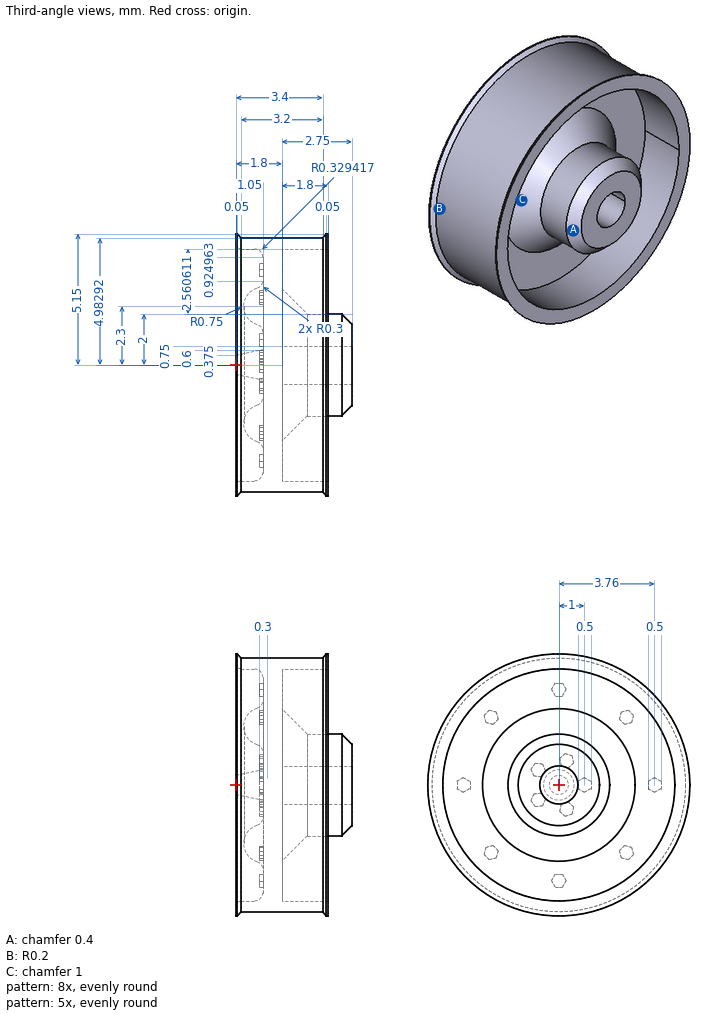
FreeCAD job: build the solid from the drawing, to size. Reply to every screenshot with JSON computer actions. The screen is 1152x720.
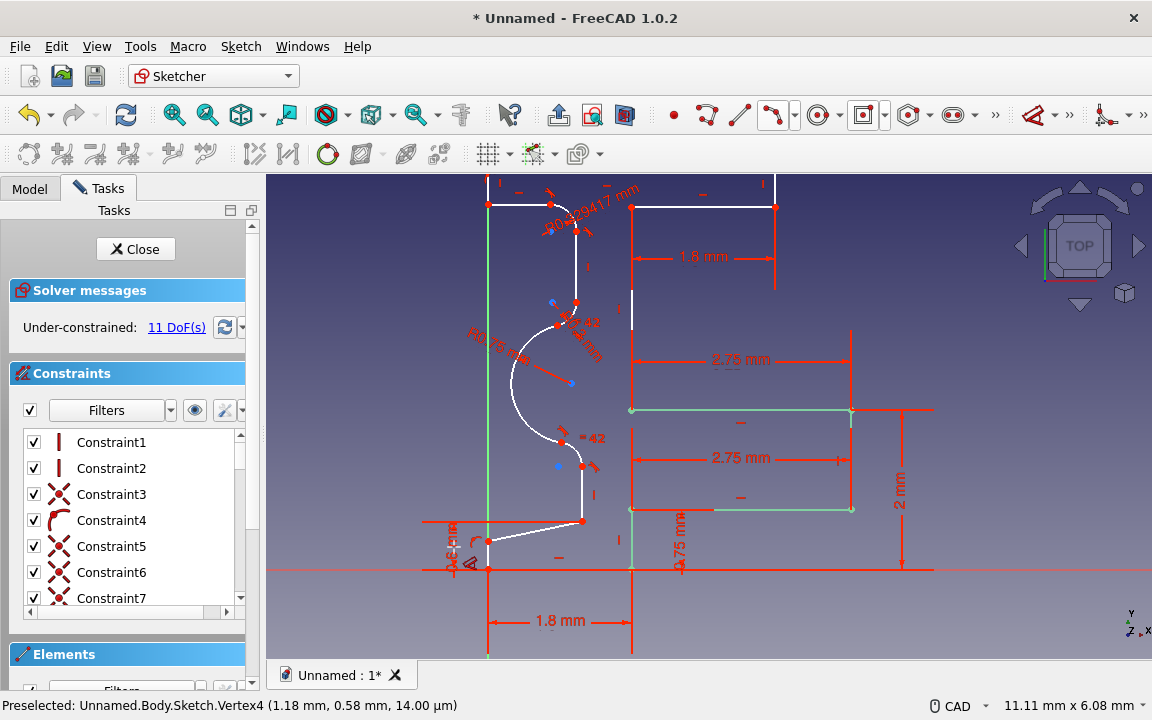
{"action": "scroll", "coordinate": [581, 523], "scroll_direction": "down", "scroll_amount": 2}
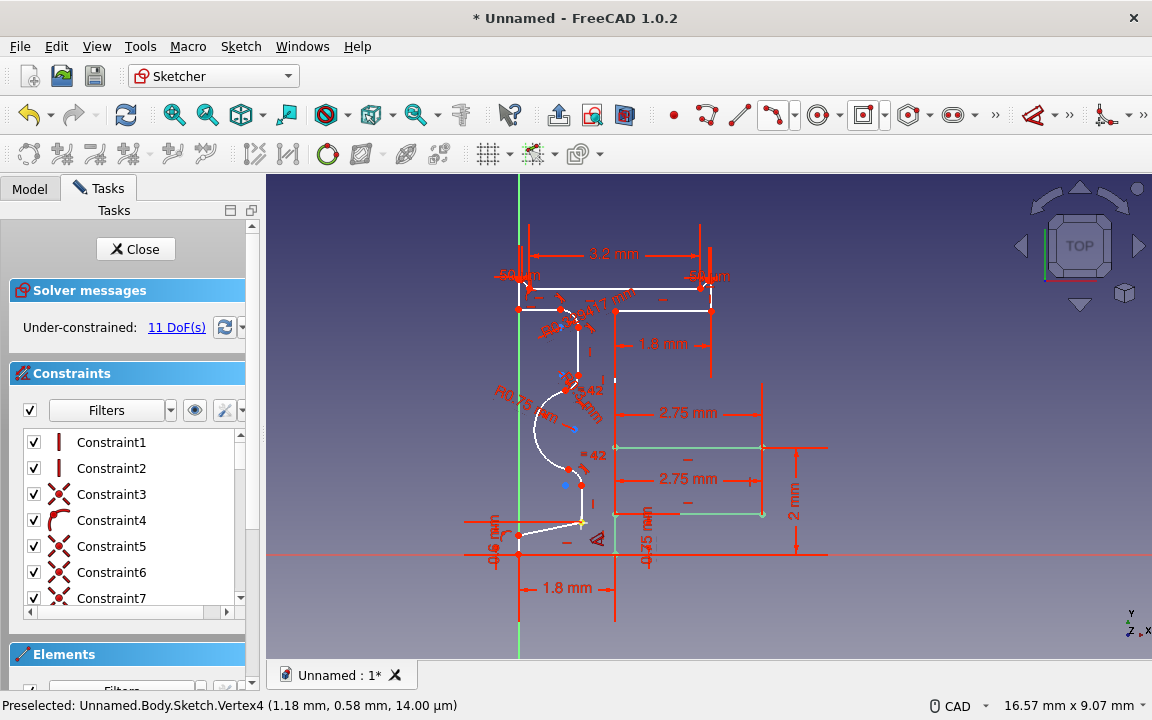
{"action": "left_click", "coordinate": [700, 289]}
{"action": "left_click", "coordinate": [651, 589]}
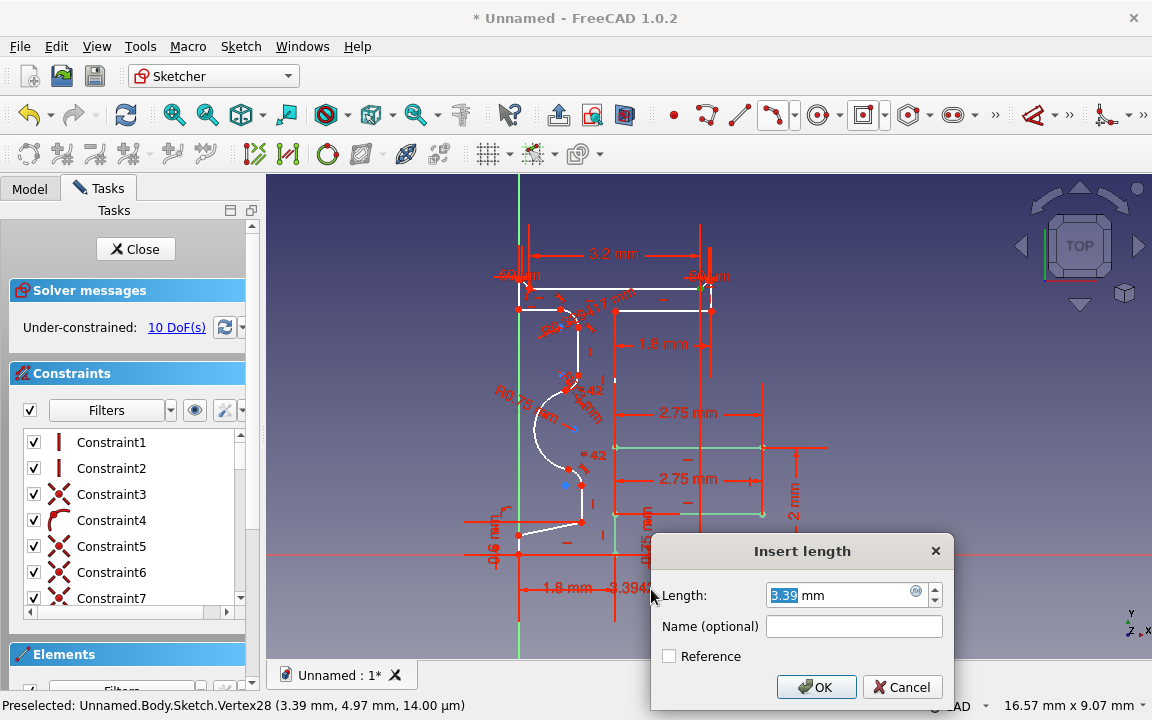
{"action": "type", "text": "3.4"}
{"action": "key", "text": "Return"}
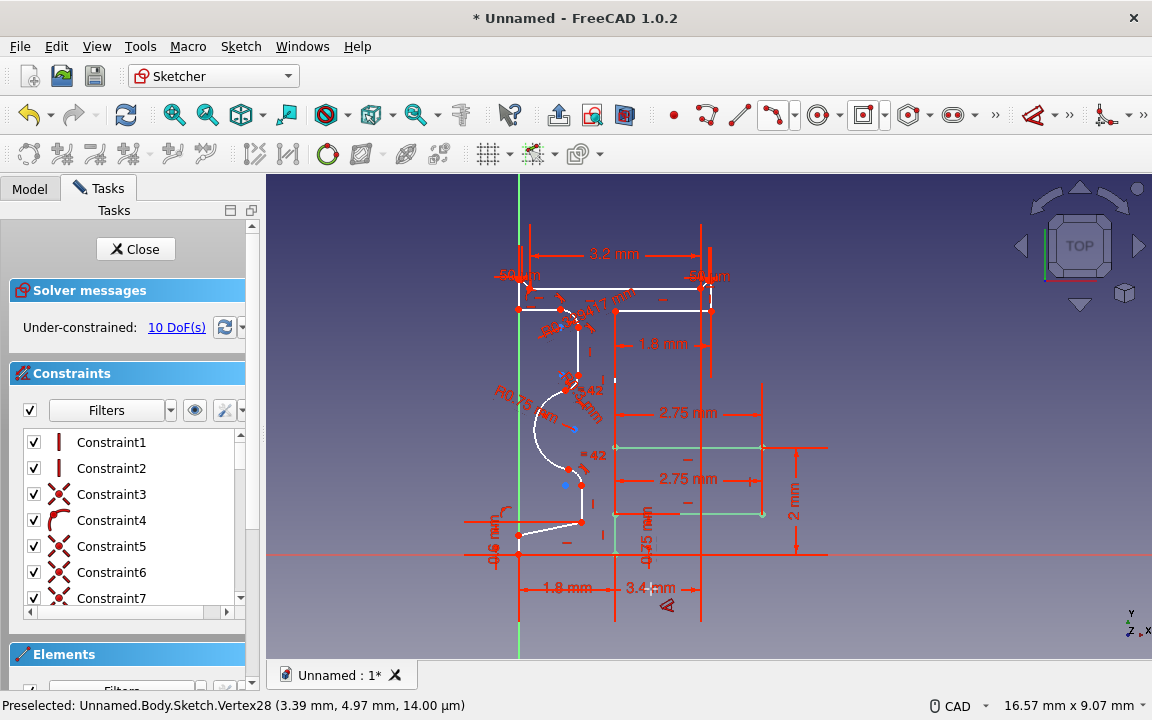
{"action": "left_click", "coordinate": [574, 430]}
{"action": "left_click", "coordinate": [485, 492]}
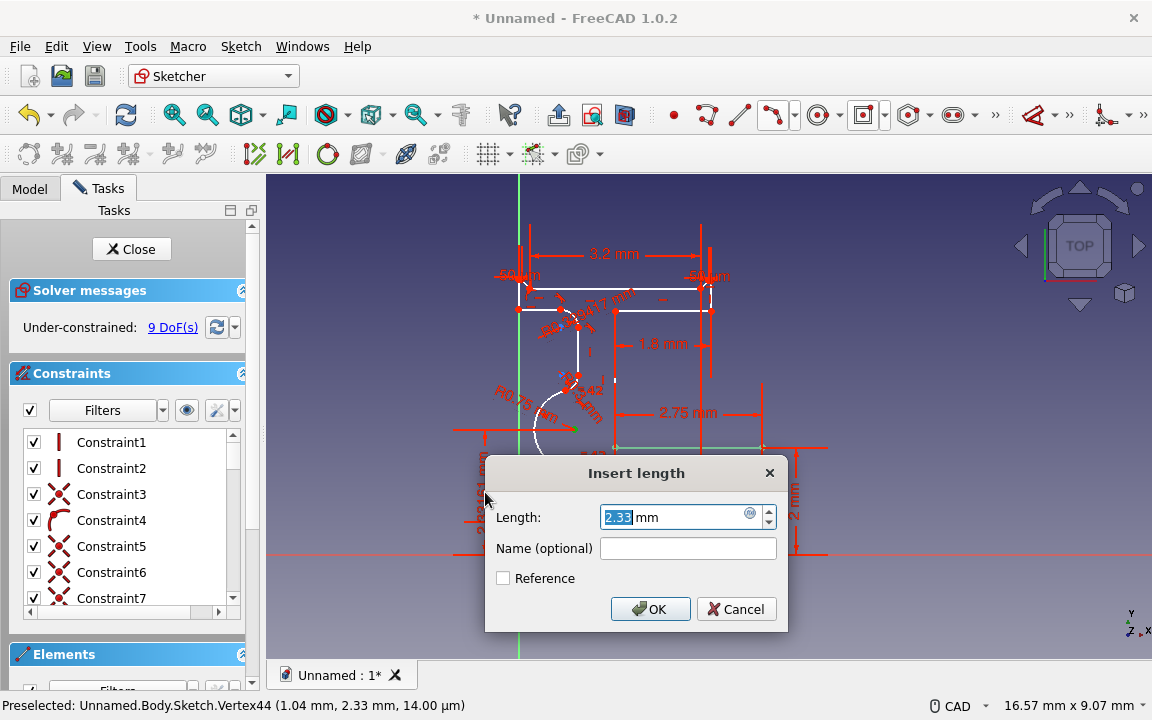
{"action": "type", "text": "2.3"}
{"action": "key", "text": "Return"}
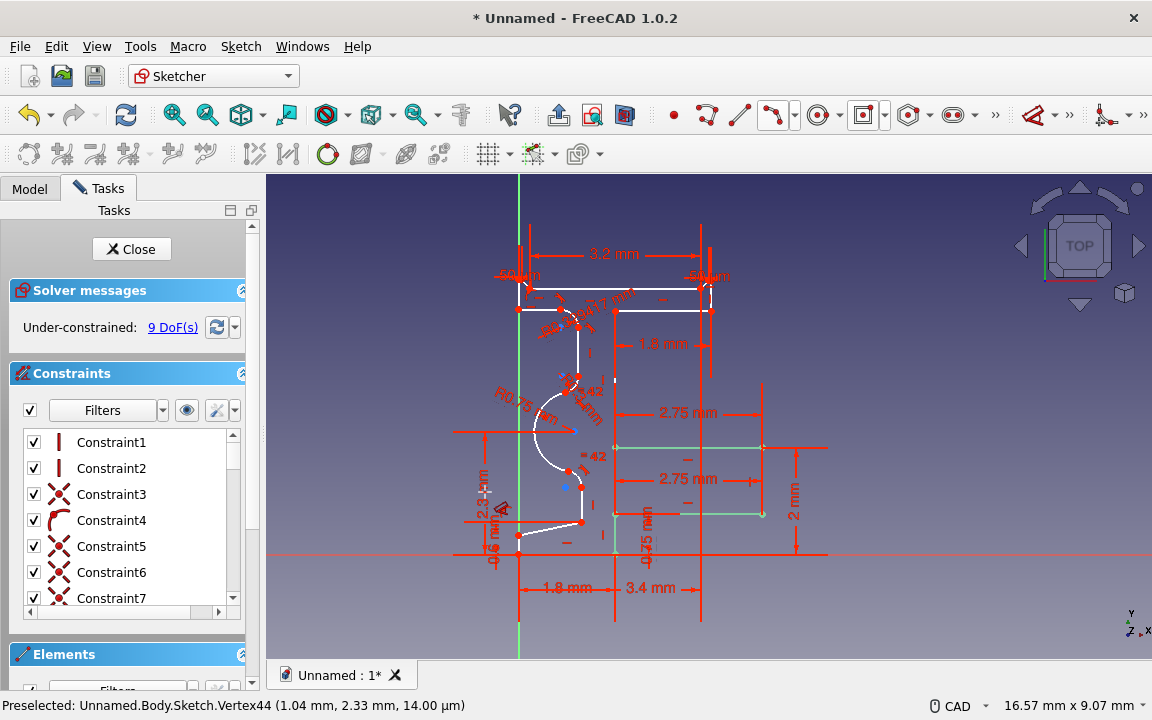
{"action": "scroll", "coordinate": [519, 545], "scroll_direction": "up", "scroll_amount": 4}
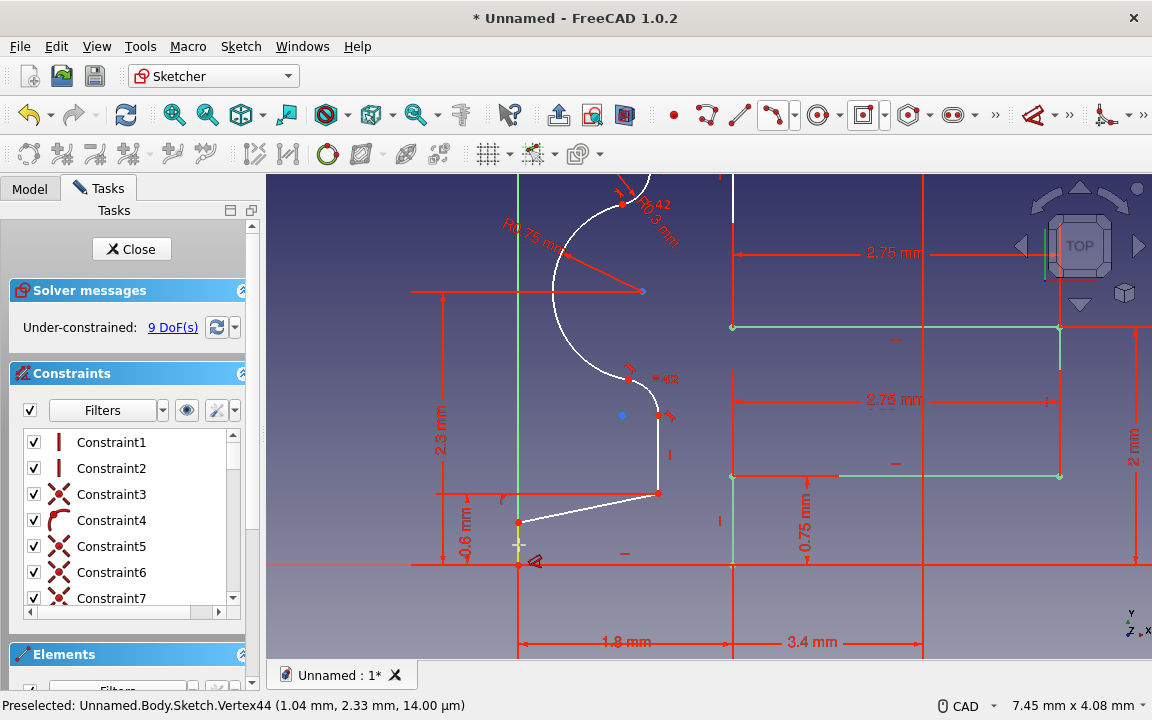
{"action": "left_click", "coordinate": [518, 544]}
{"action": "left_click", "coordinate": [552, 544]}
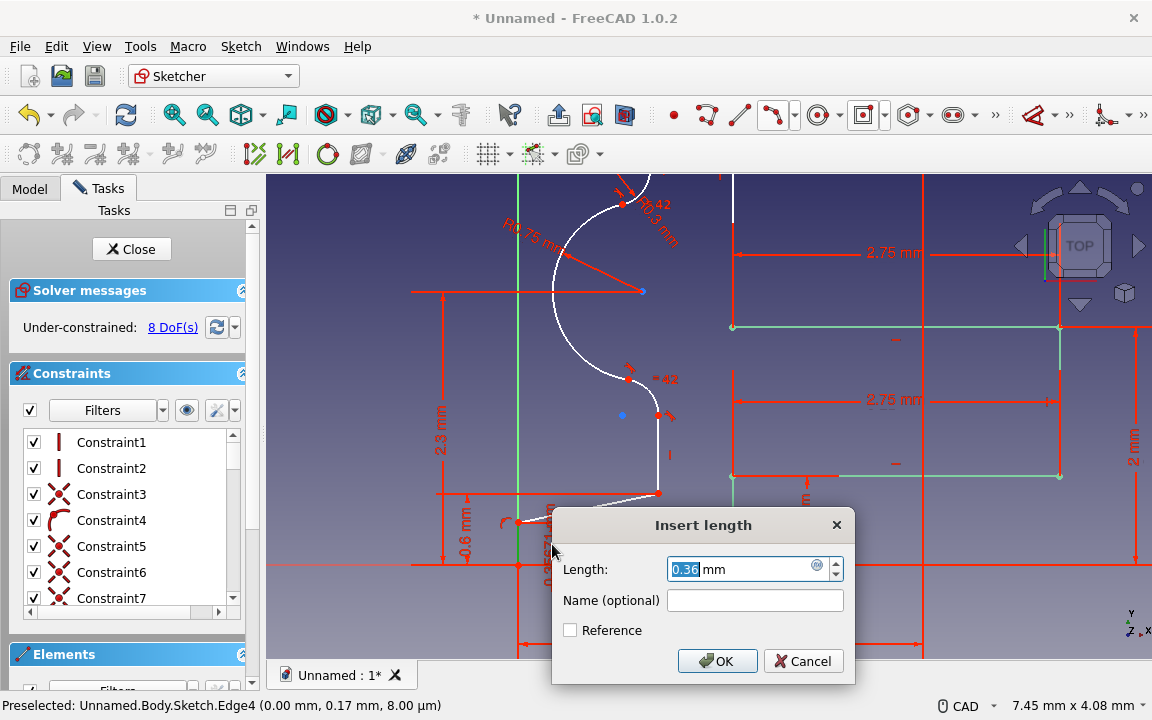
{"action": "type", "text": "0.375"}
{"action": "key", "text": "Return"}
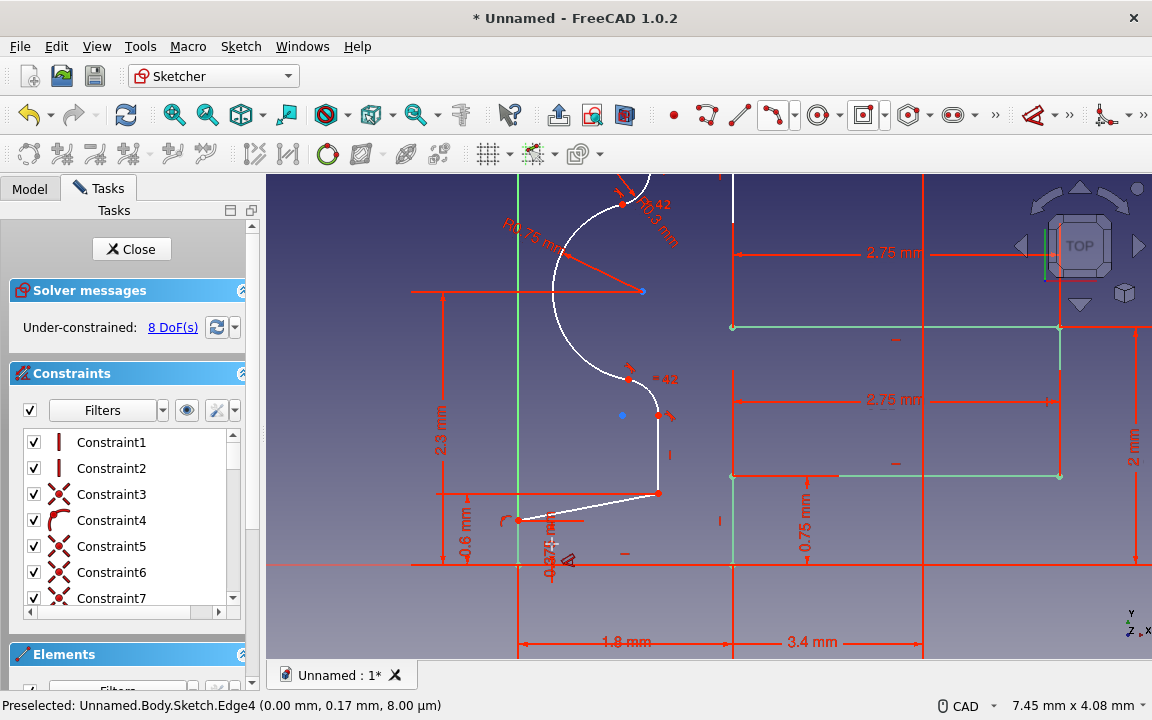
{"action": "scroll", "coordinate": [519, 545], "scroll_direction": "down", "scroll_amount": 4}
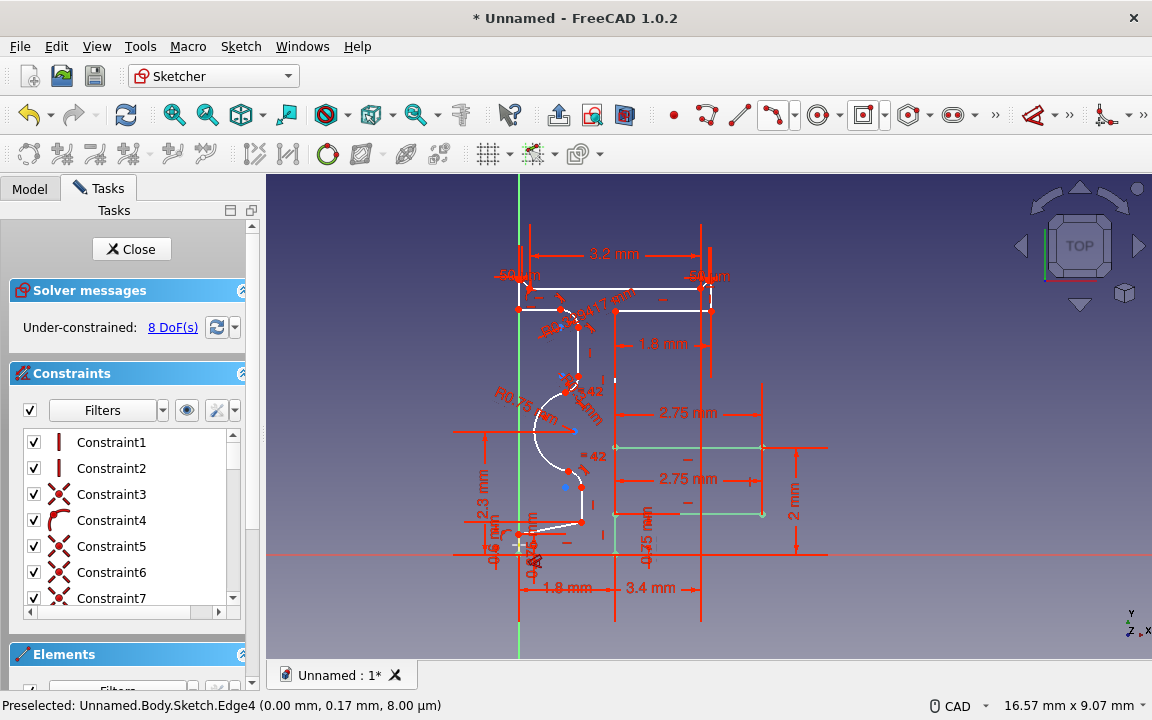
{"action": "left_click", "coordinate": [578, 328]}
{"action": "left_click", "coordinate": [548, 613]}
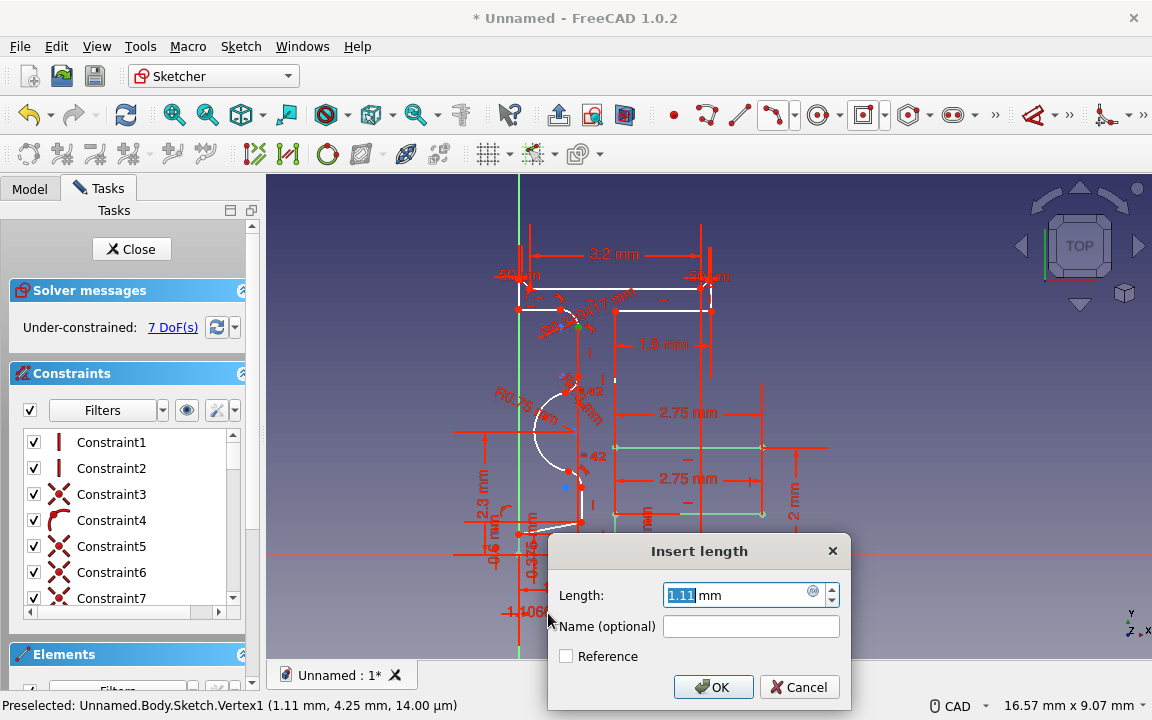
{"action": "type", "text": "1.05"}
{"action": "key", "text": "Return"}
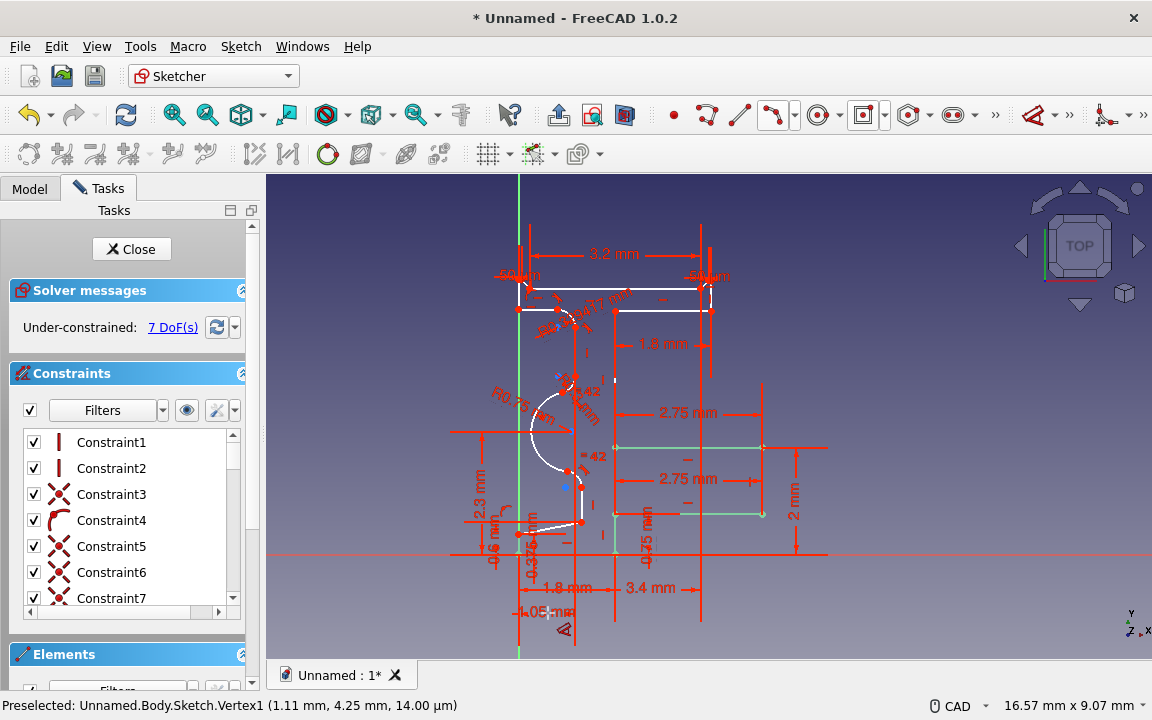
{"action": "left_click", "coordinate": [582, 487]}
{"action": "left_click", "coordinate": [565, 453]}